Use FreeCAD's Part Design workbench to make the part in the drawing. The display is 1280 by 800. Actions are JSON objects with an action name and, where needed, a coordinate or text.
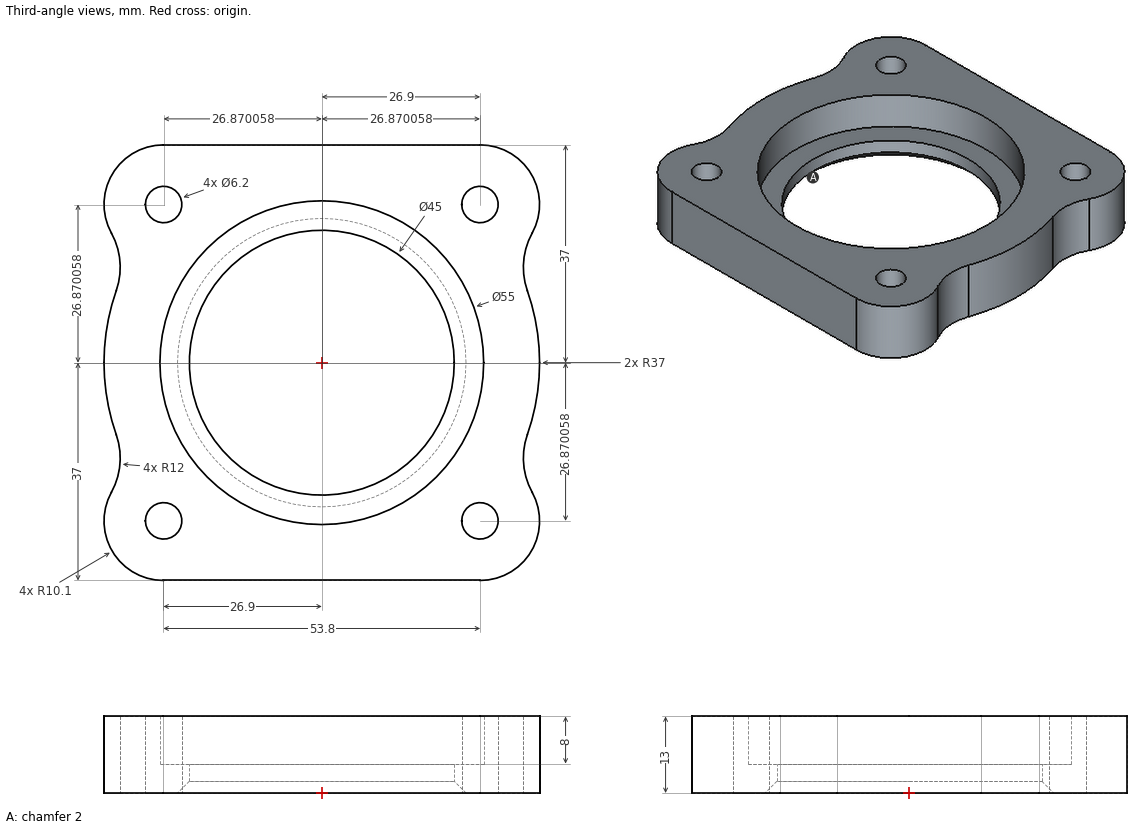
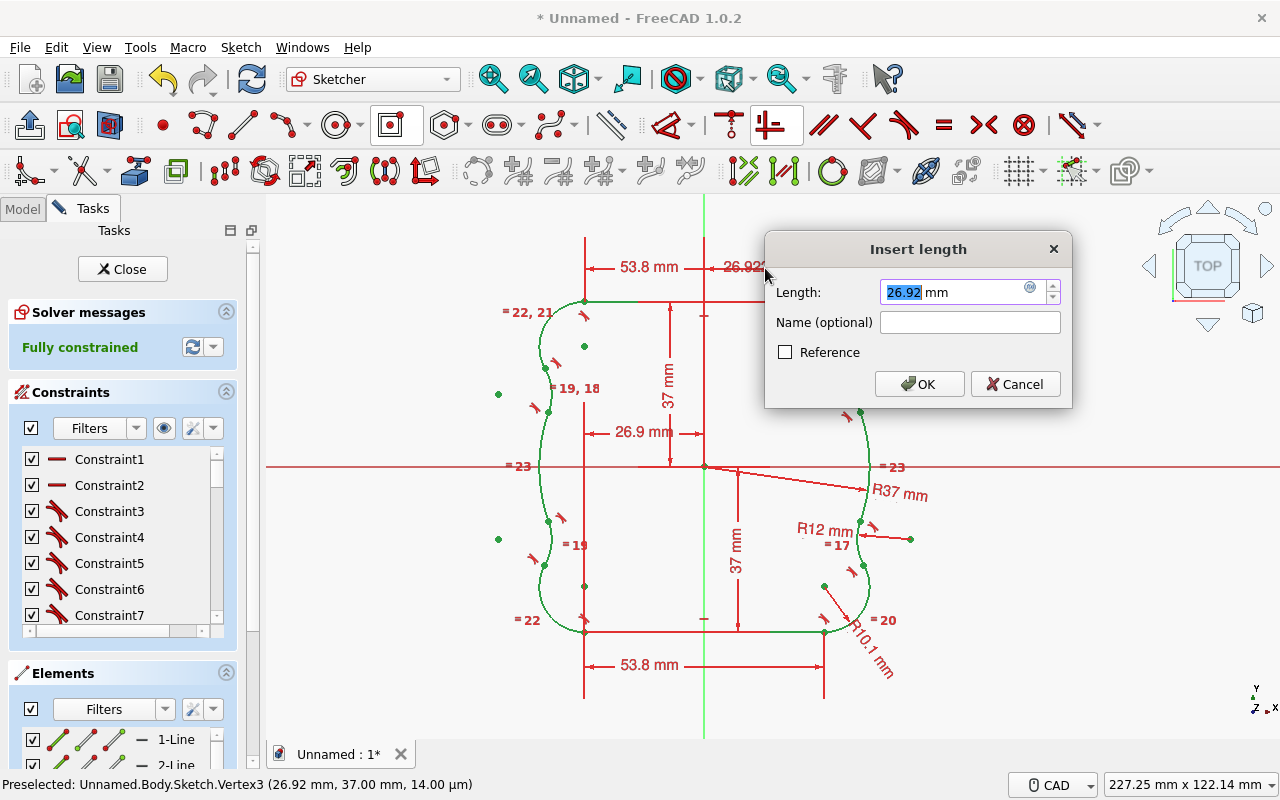
{"action": "type", "text": "26.9"}
{"action": "key", "text": "Return"}
{"action": "key", "text": "Escape"}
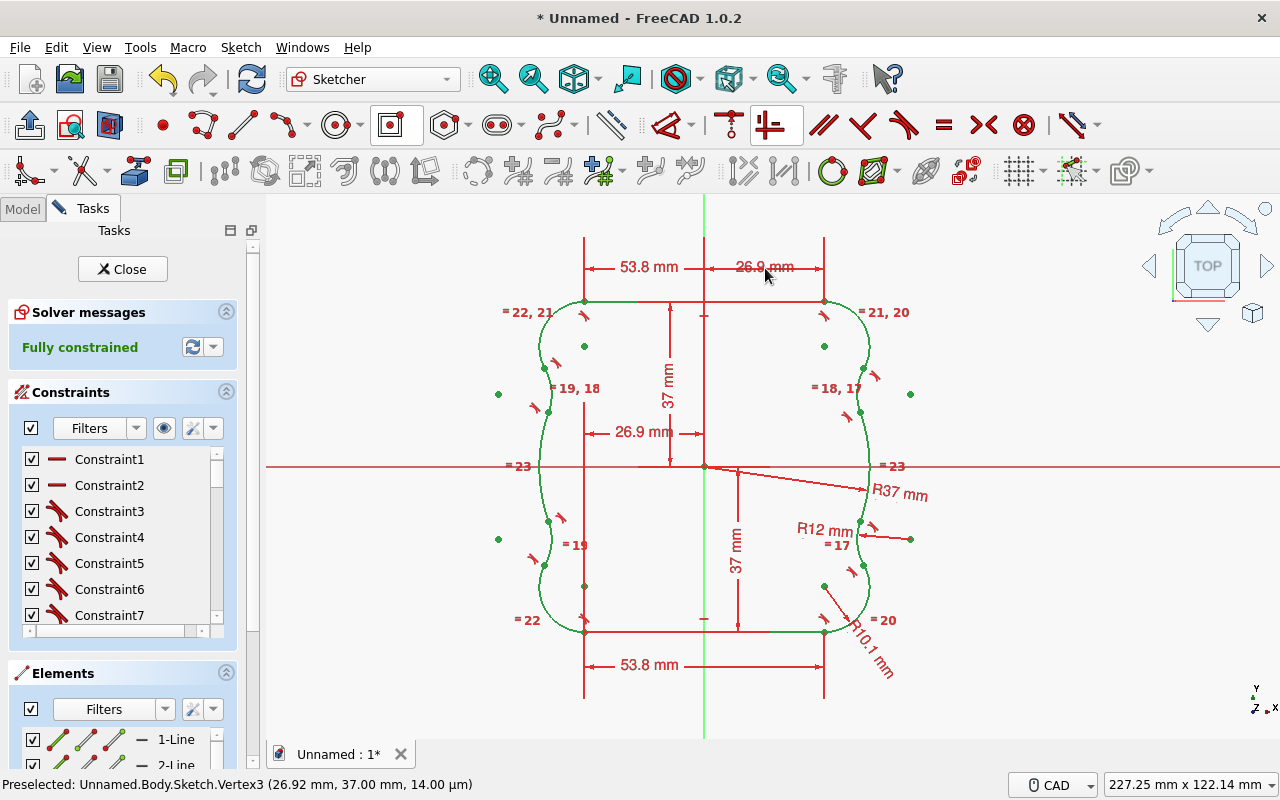
{"action": "left_click", "coordinate": [123, 269]}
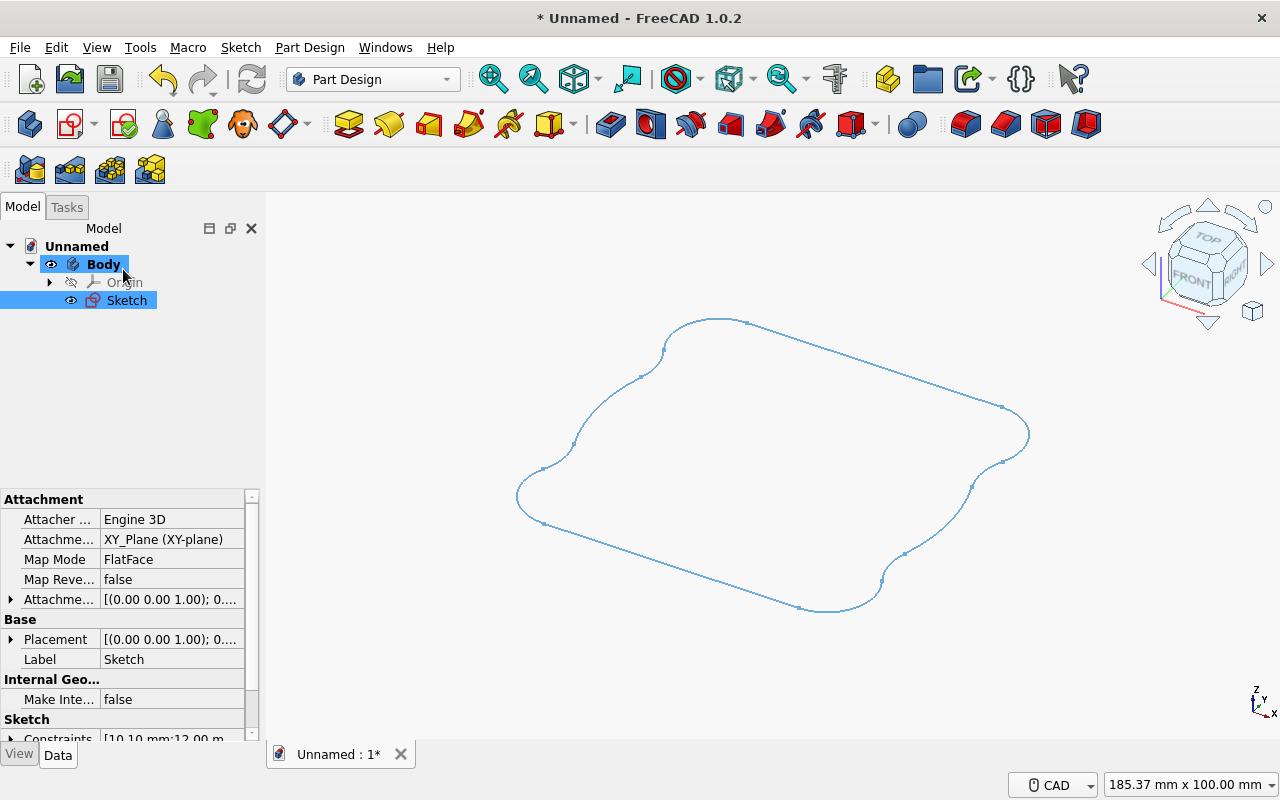
{"action": "left_click", "coordinate": [350, 124]}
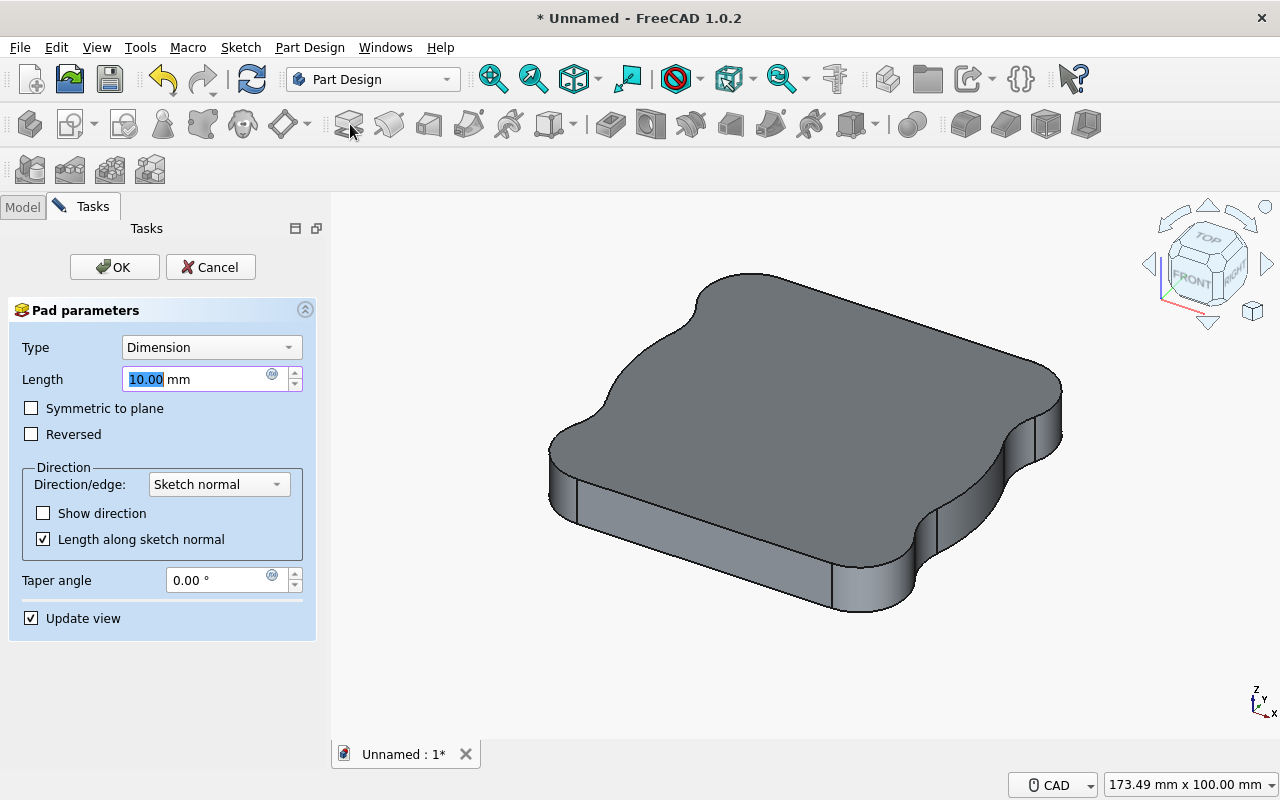
{"action": "type", "text": "13"}
{"action": "key", "text": "Tab"}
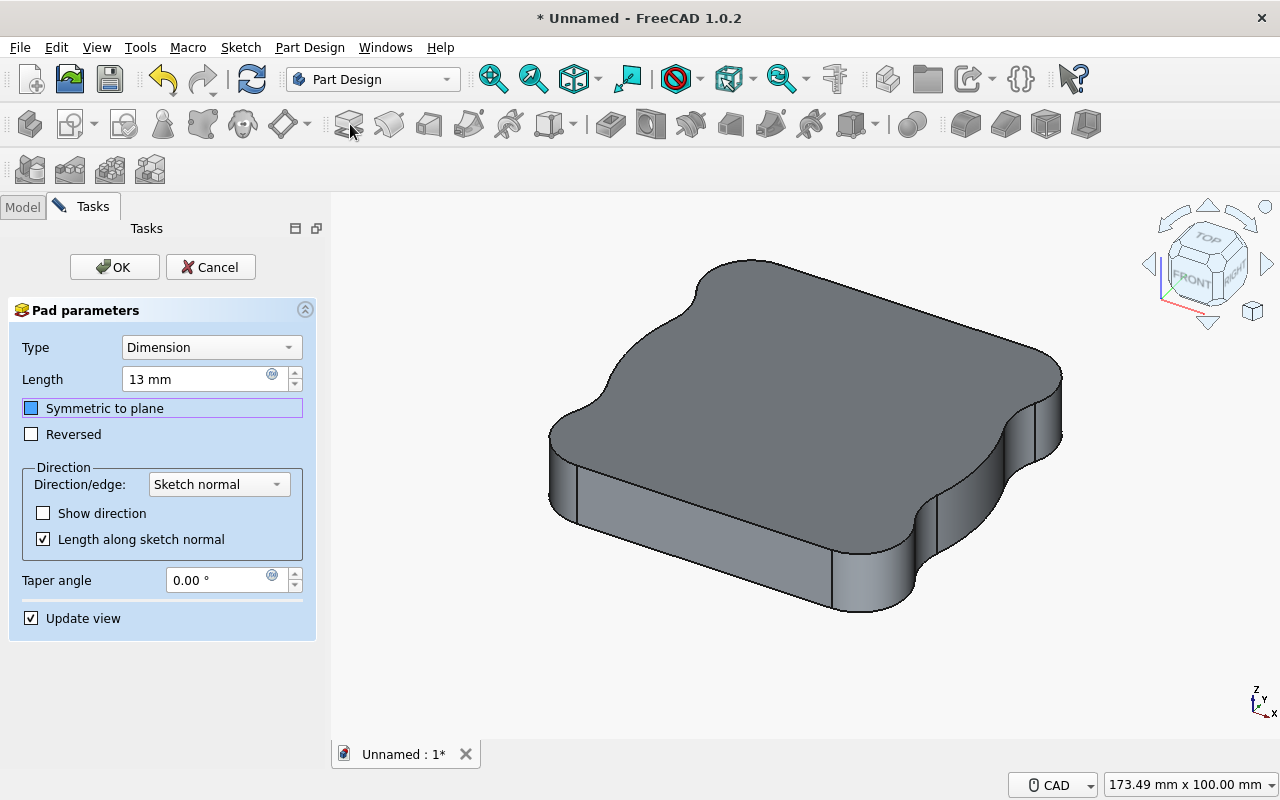
{"action": "left_click", "coordinate": [115, 267]}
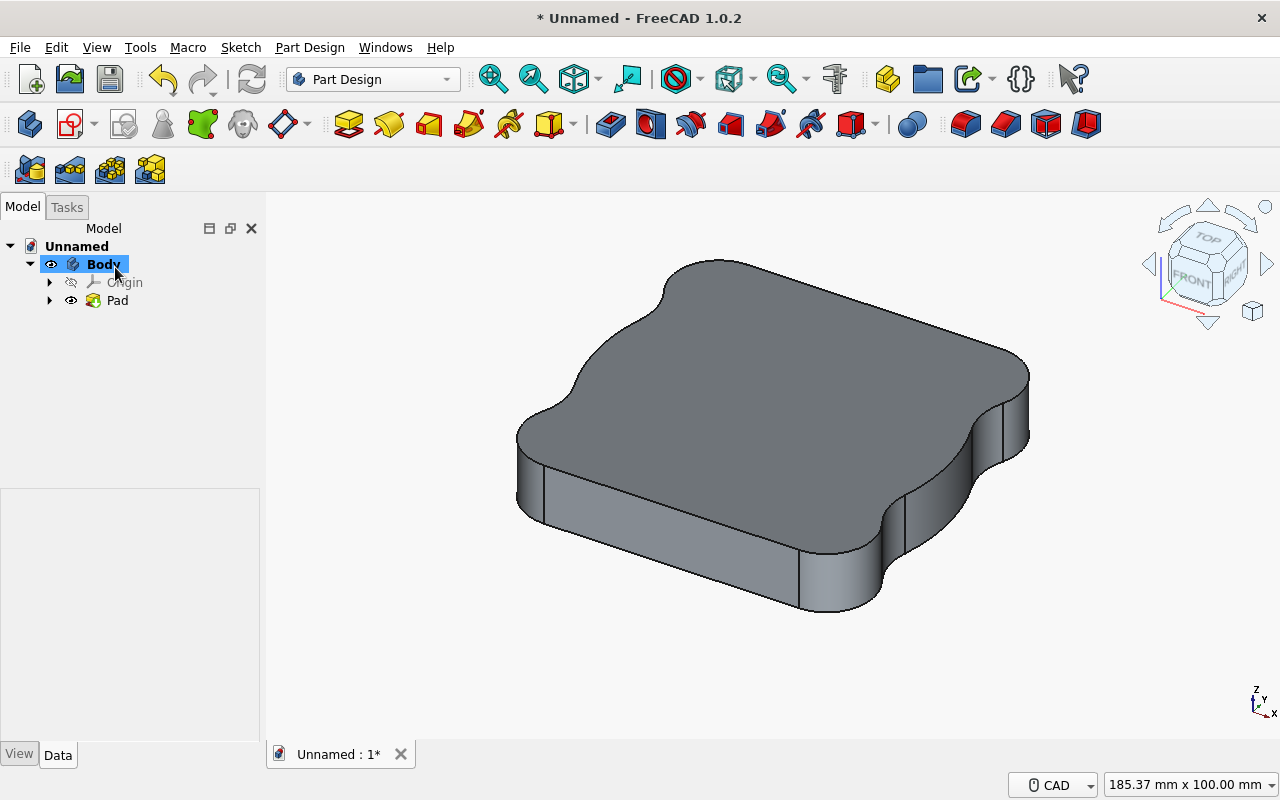
{"action": "left_click", "coordinate": [773, 406]}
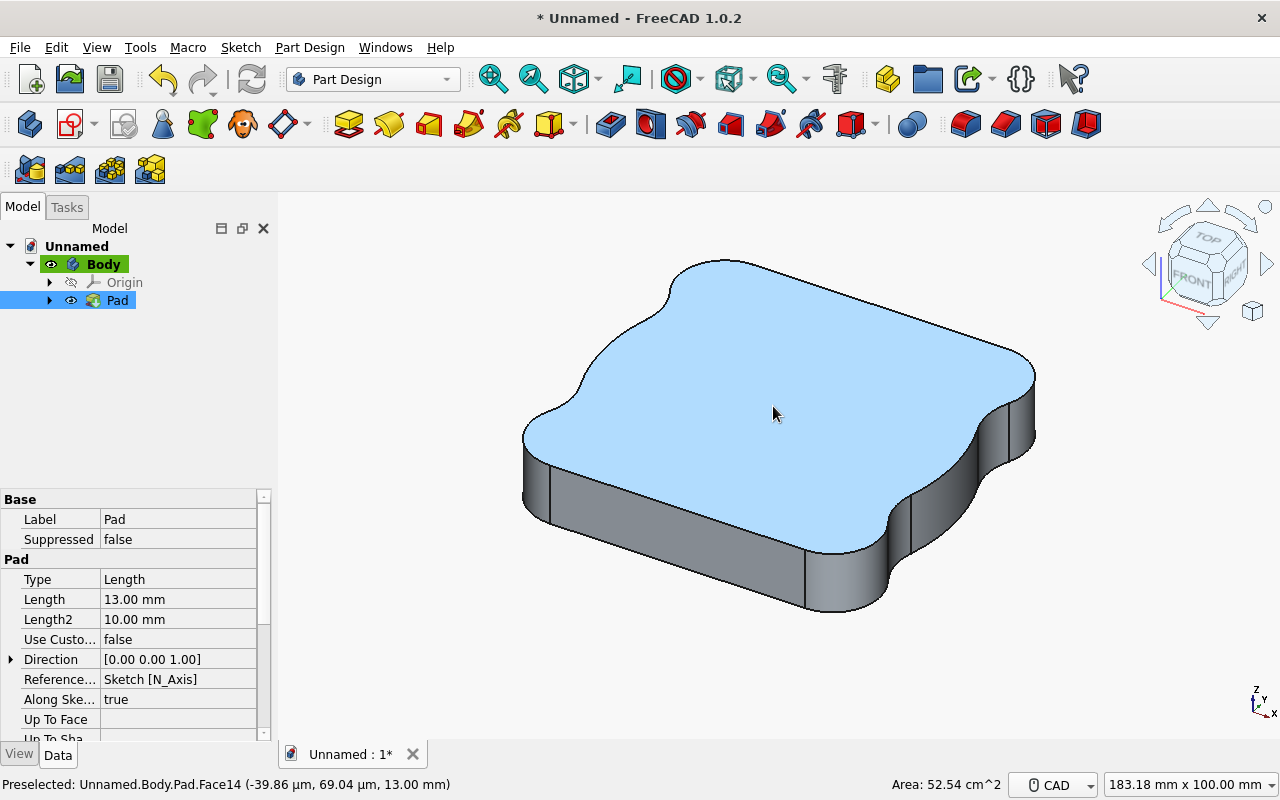
{"action": "left_click", "coordinate": [70, 124]}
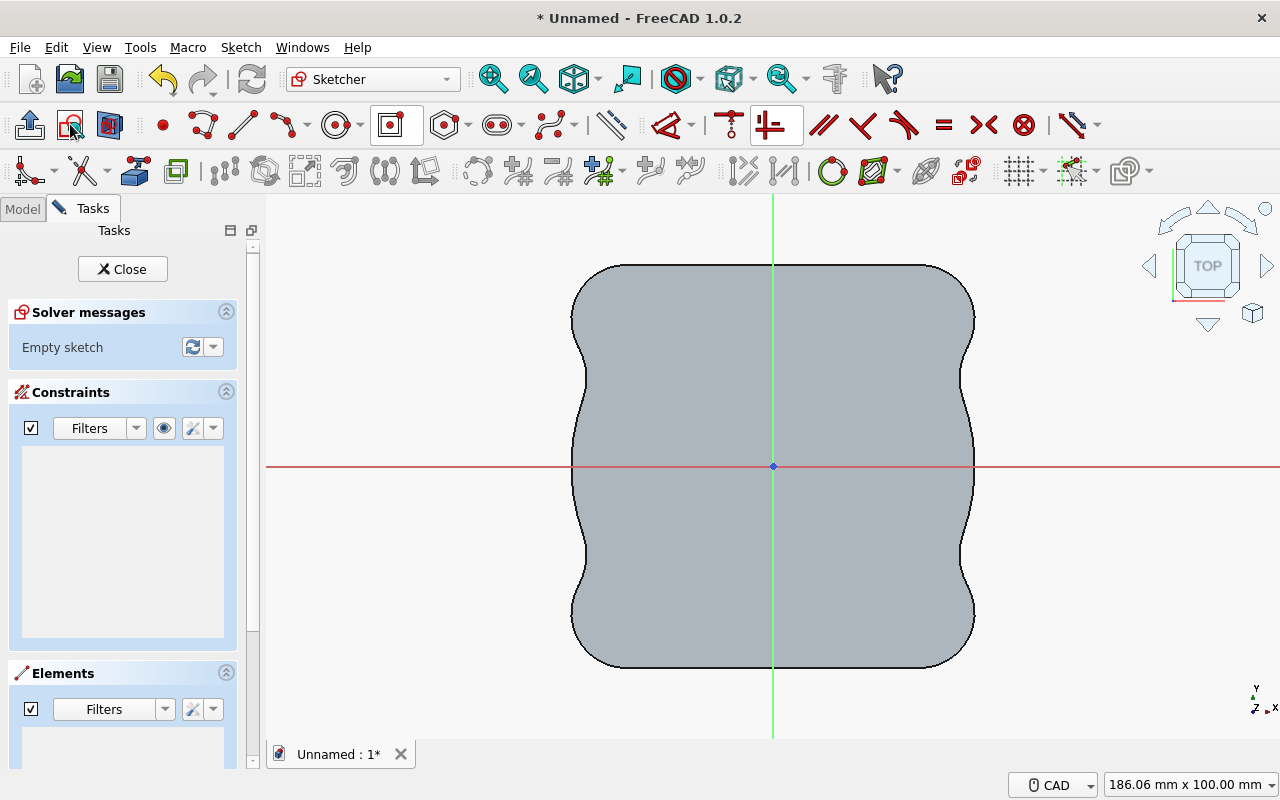
{"action": "key", "text": "g c"}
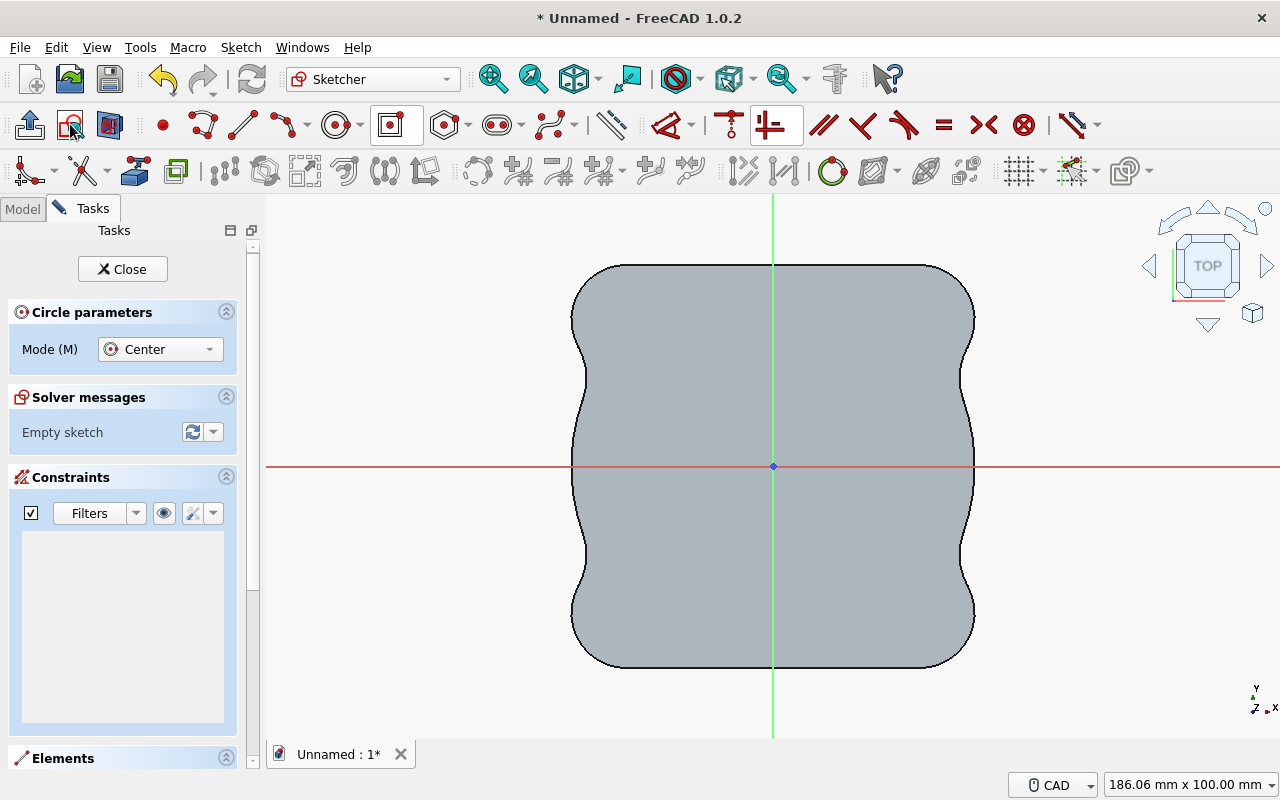
{"action": "scroll", "coordinate": [627, 320], "scroll_direction": "up", "scroll_amount": 2}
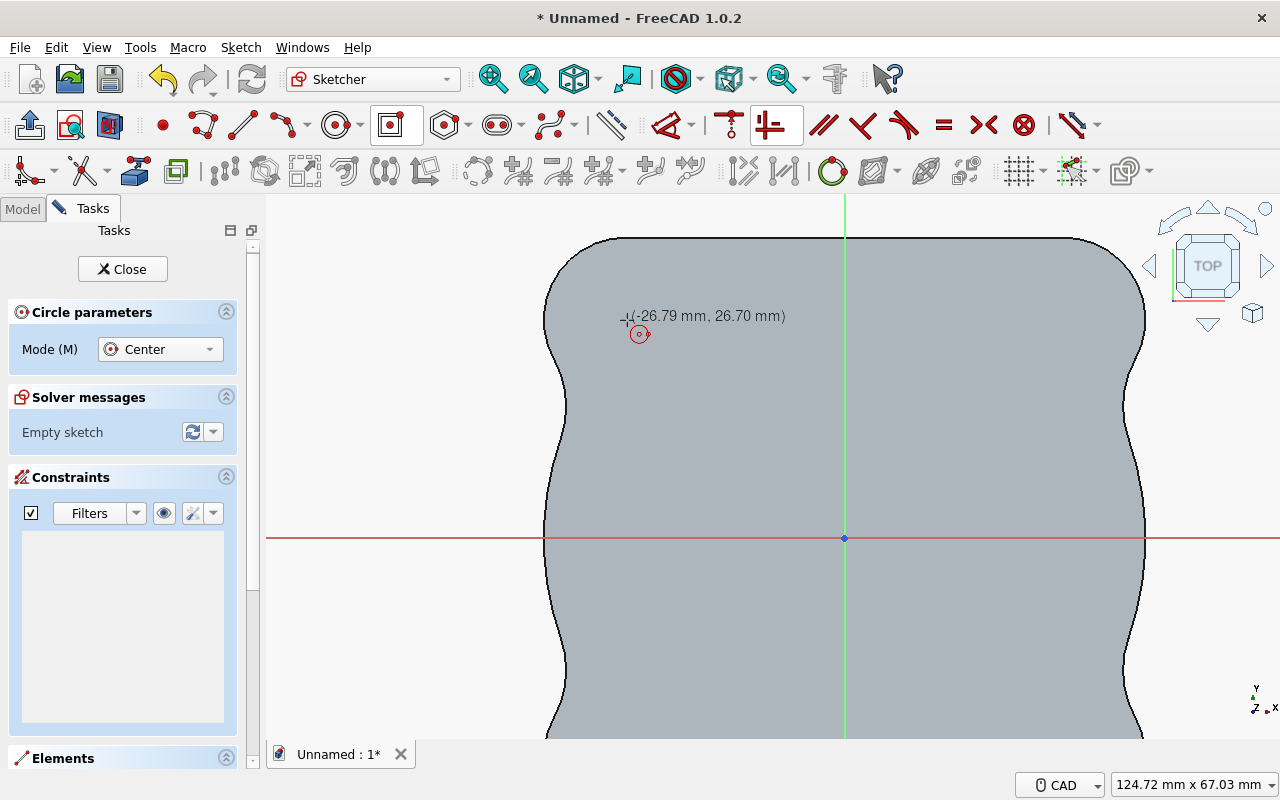
{"action": "left_click", "coordinate": [626, 320]}
{"action": "left_click", "coordinate": [644, 302]}